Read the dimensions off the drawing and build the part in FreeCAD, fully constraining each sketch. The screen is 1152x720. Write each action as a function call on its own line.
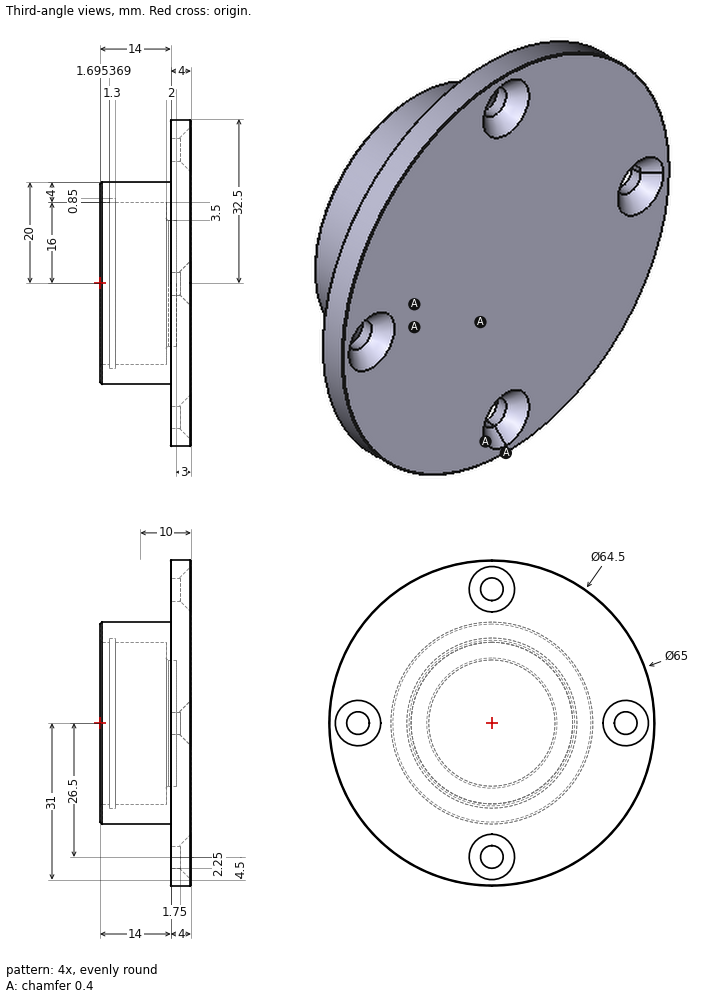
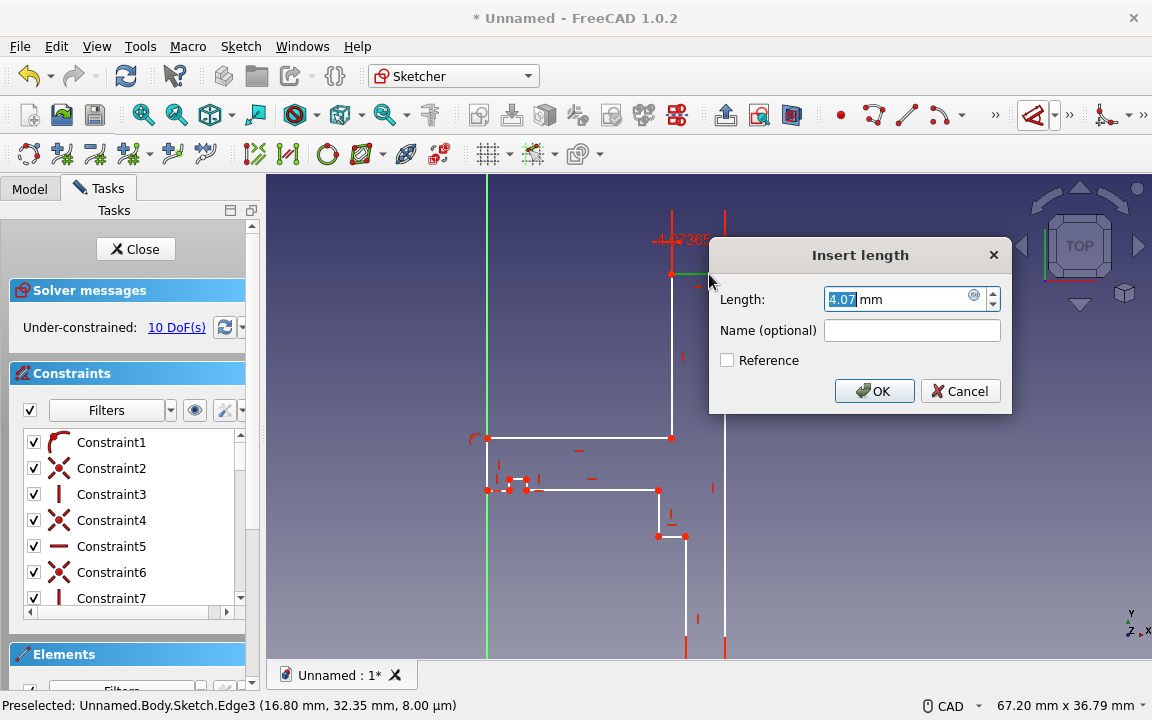
text(4)
key(Return)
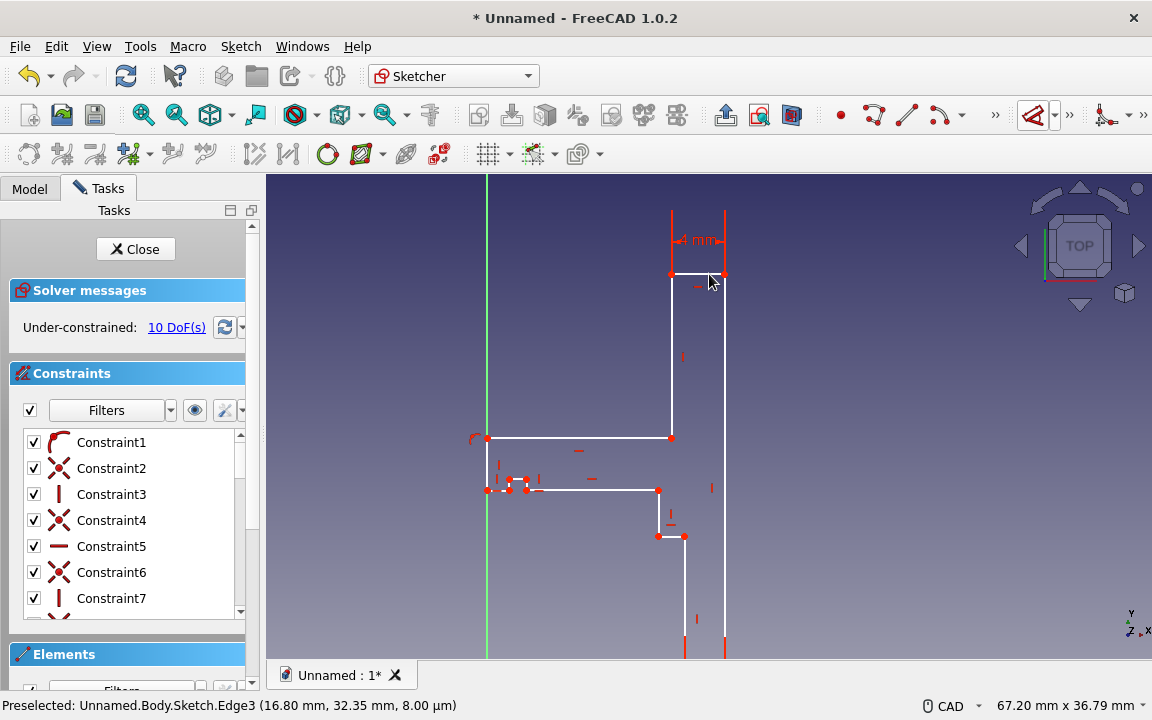
click(487, 454)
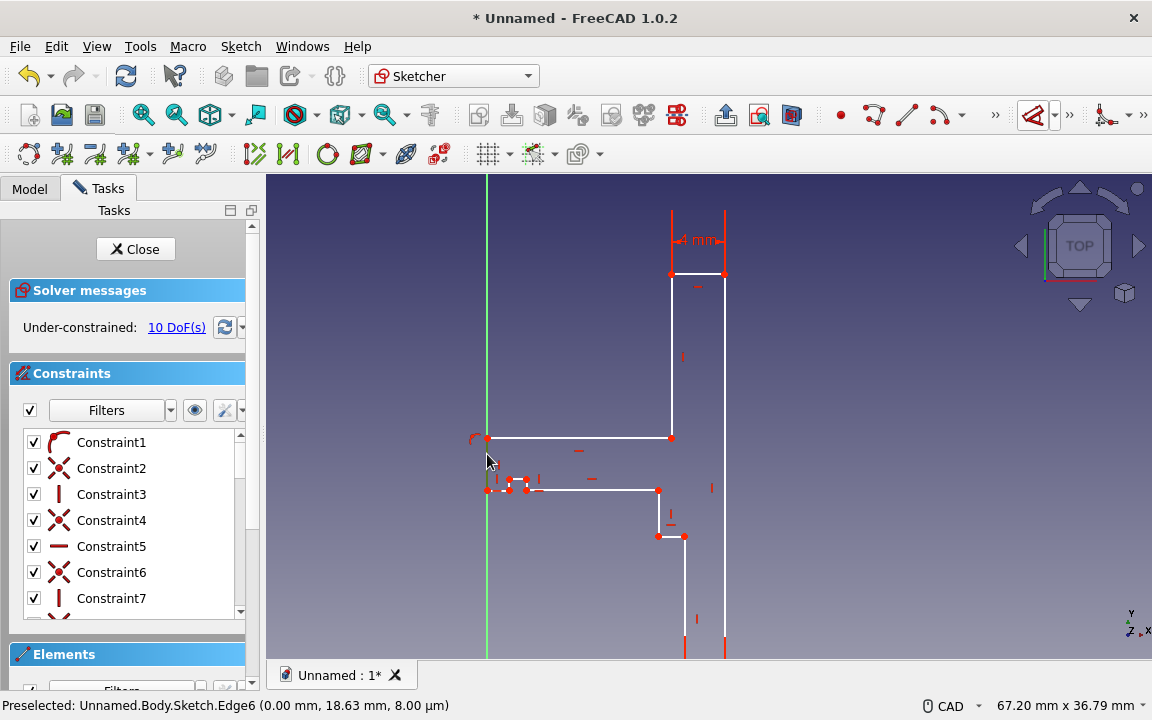
key(i)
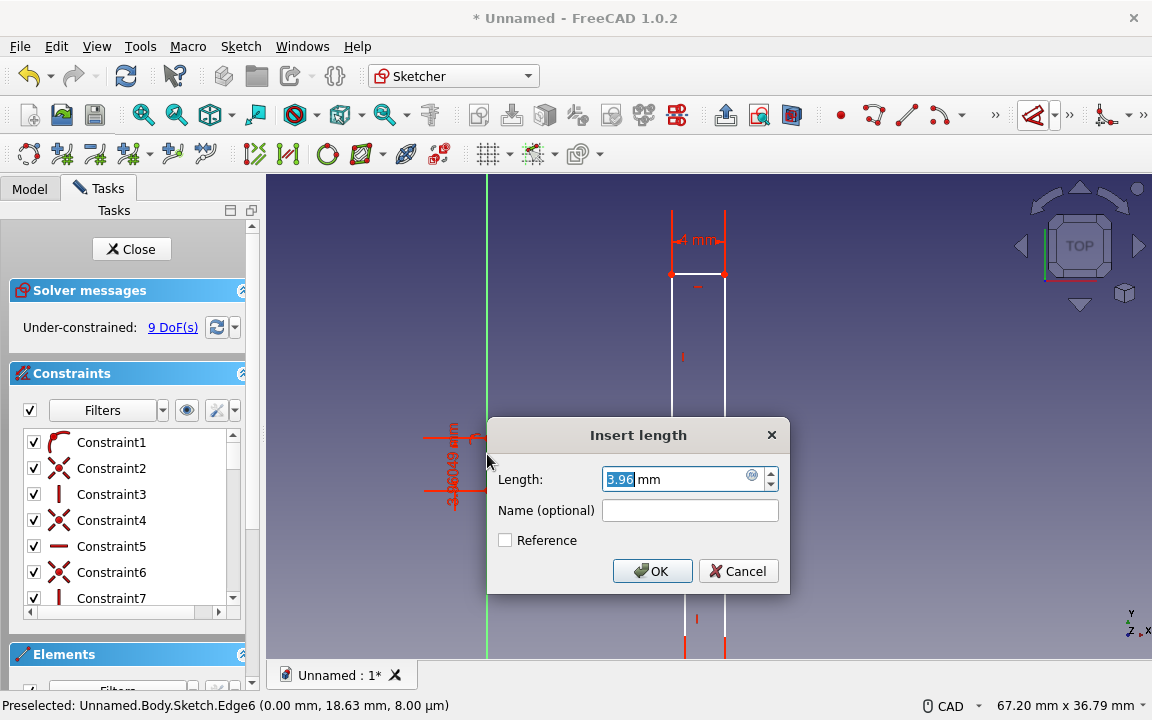
text(4)
key(Return)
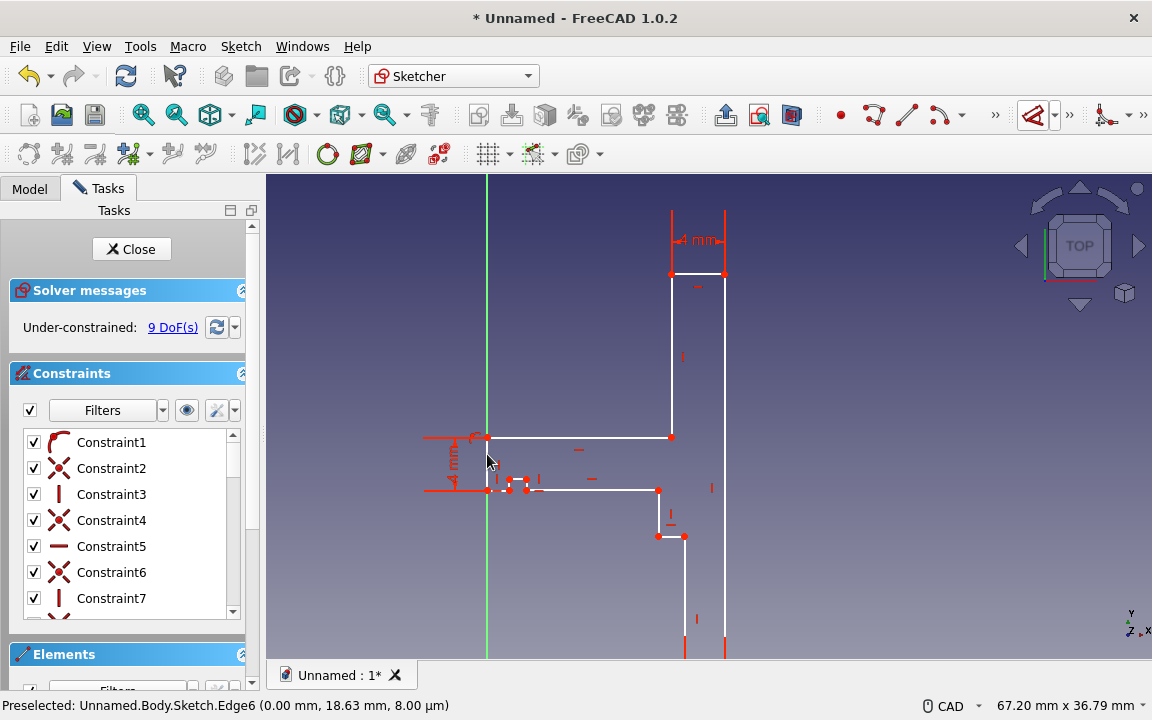
scroll(669, 537, up, 3)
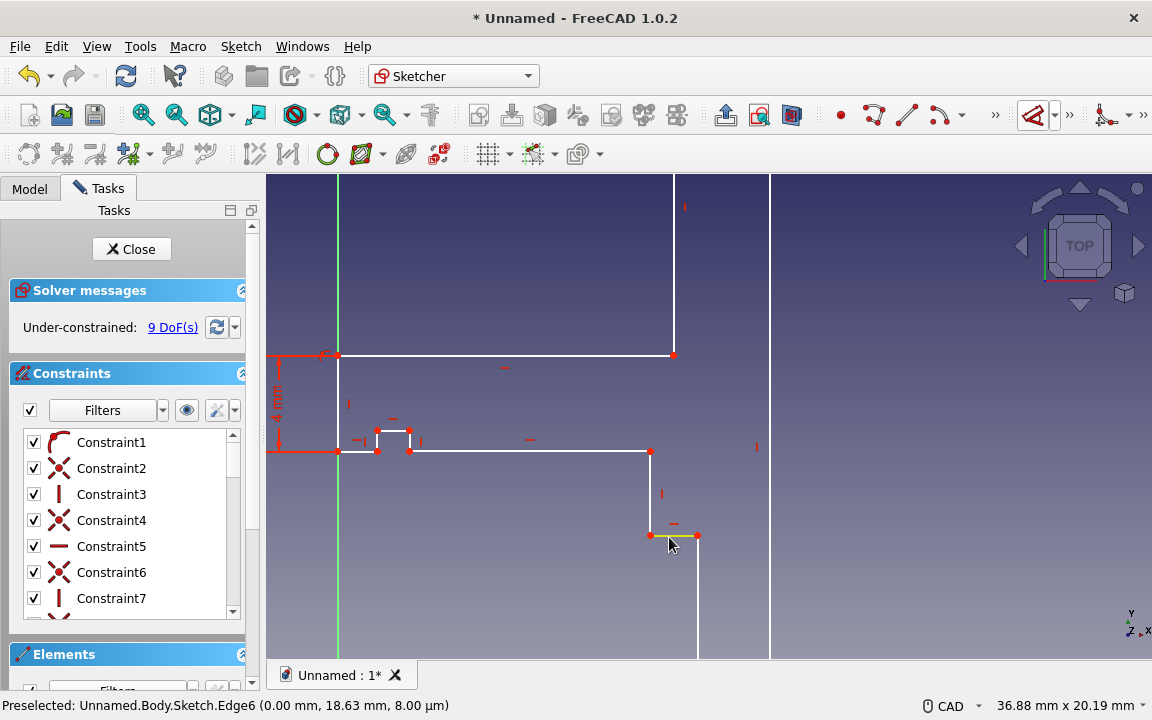
click(669, 536)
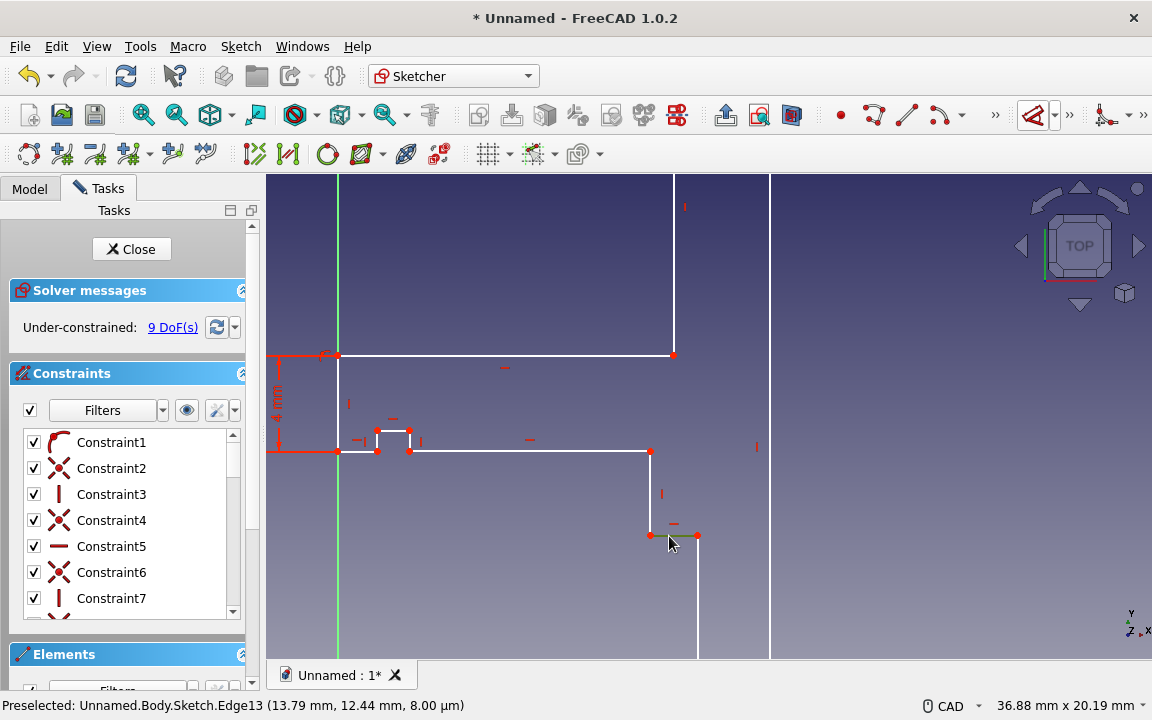
key(l)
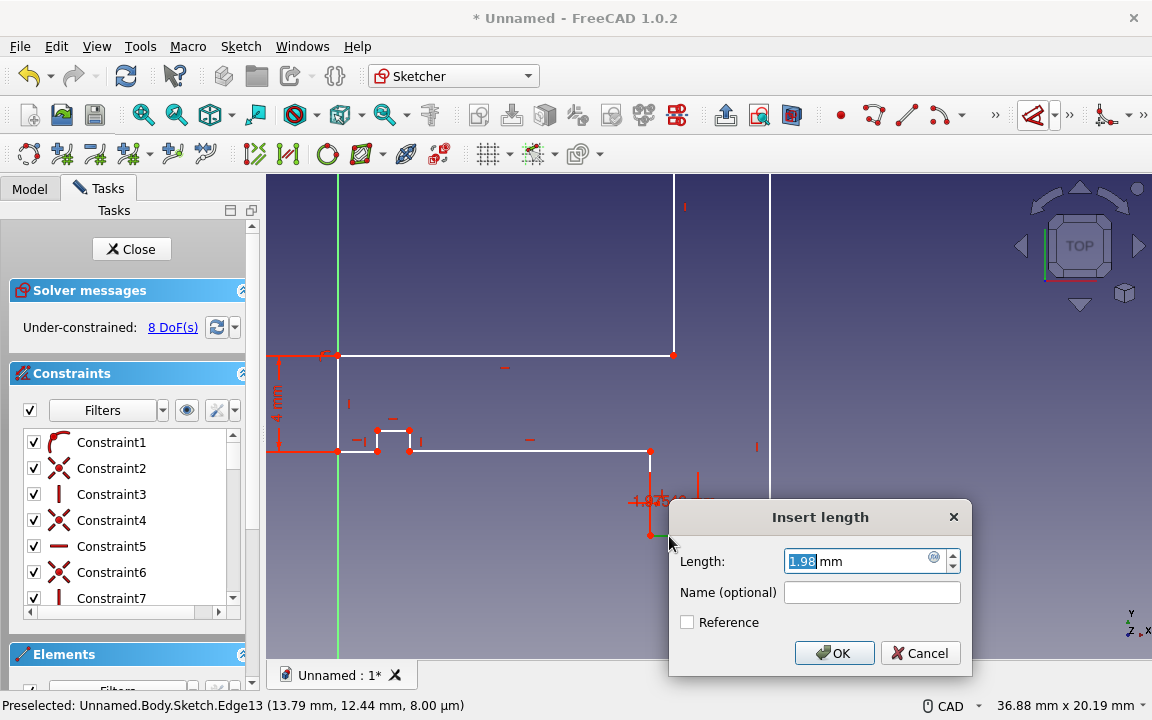
text(2)
key(Return)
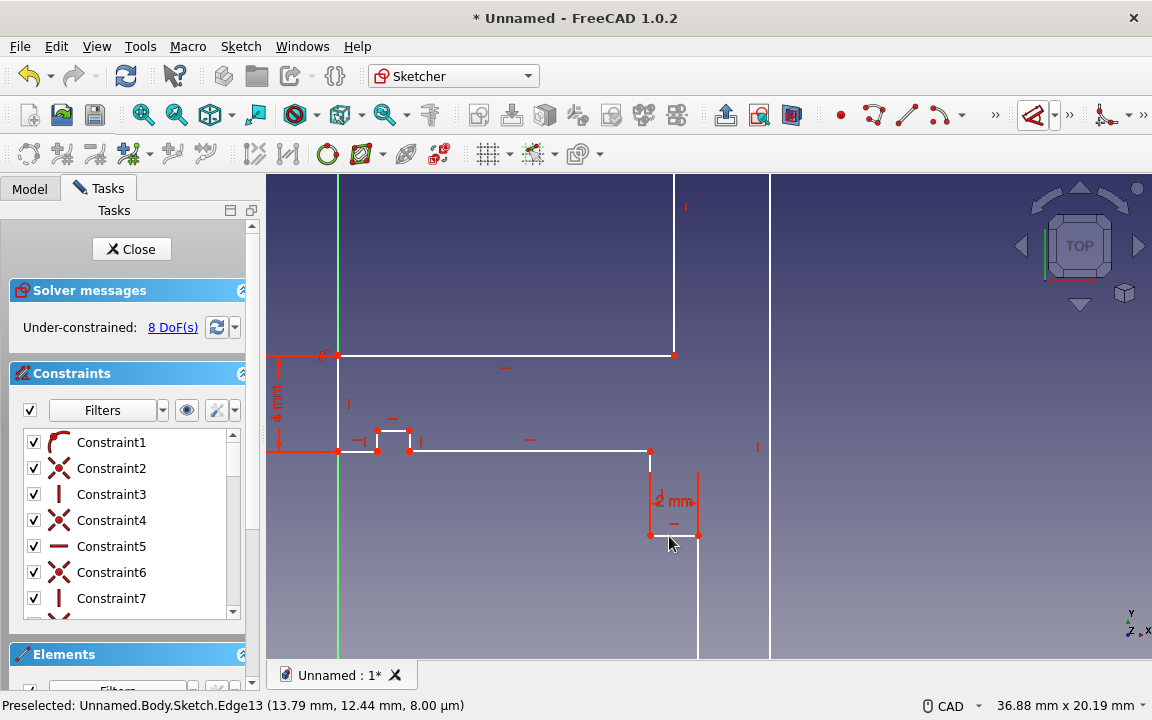
click(573, 356)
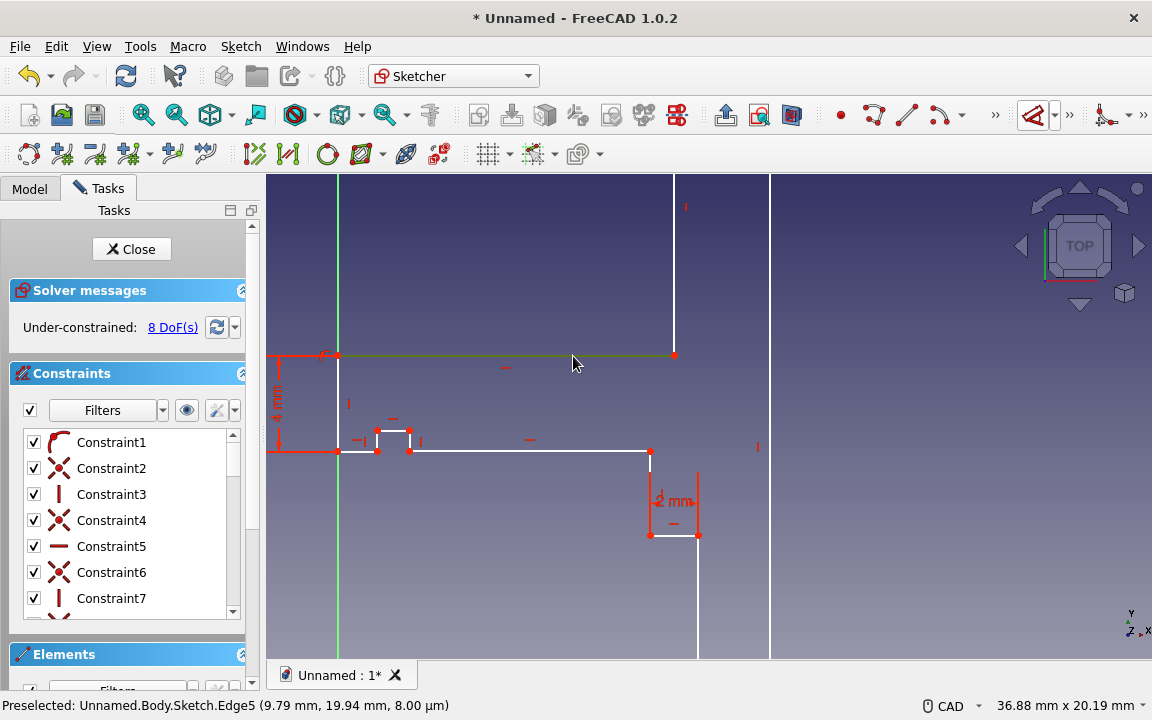
click(1054, 116)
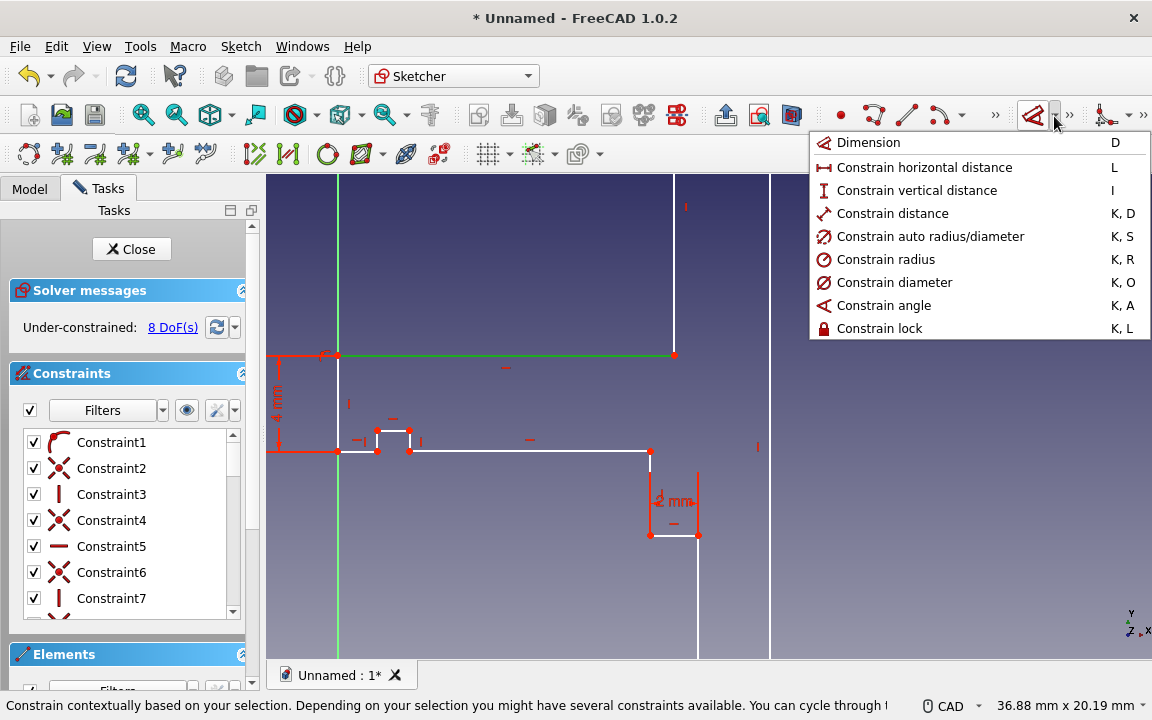
click(980, 168)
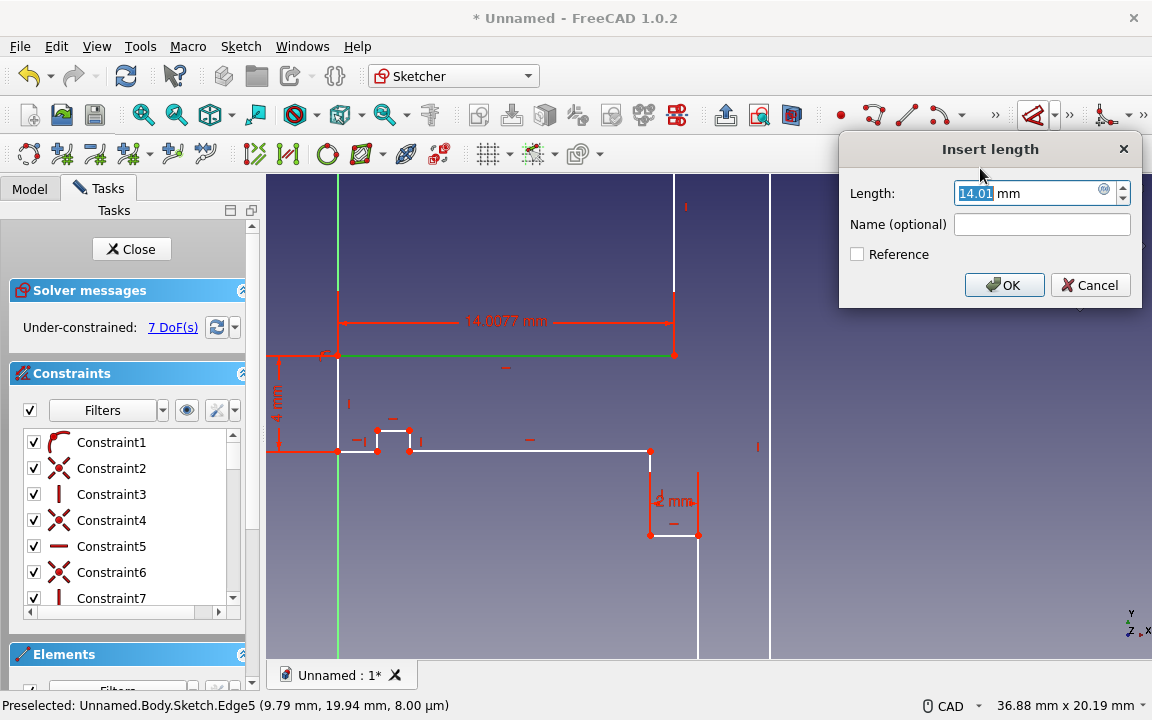
text(14)
key(Return)